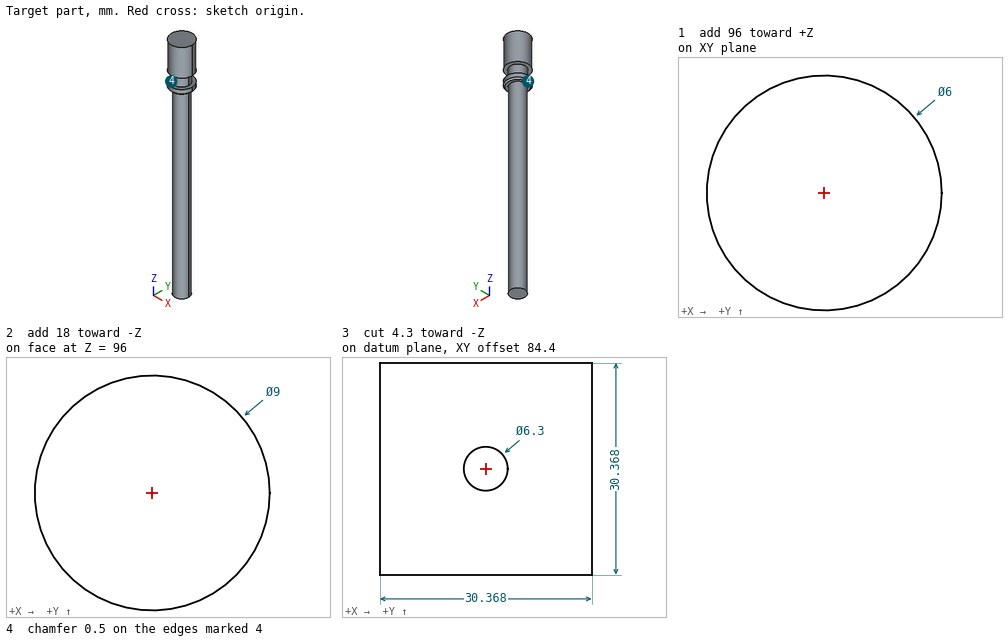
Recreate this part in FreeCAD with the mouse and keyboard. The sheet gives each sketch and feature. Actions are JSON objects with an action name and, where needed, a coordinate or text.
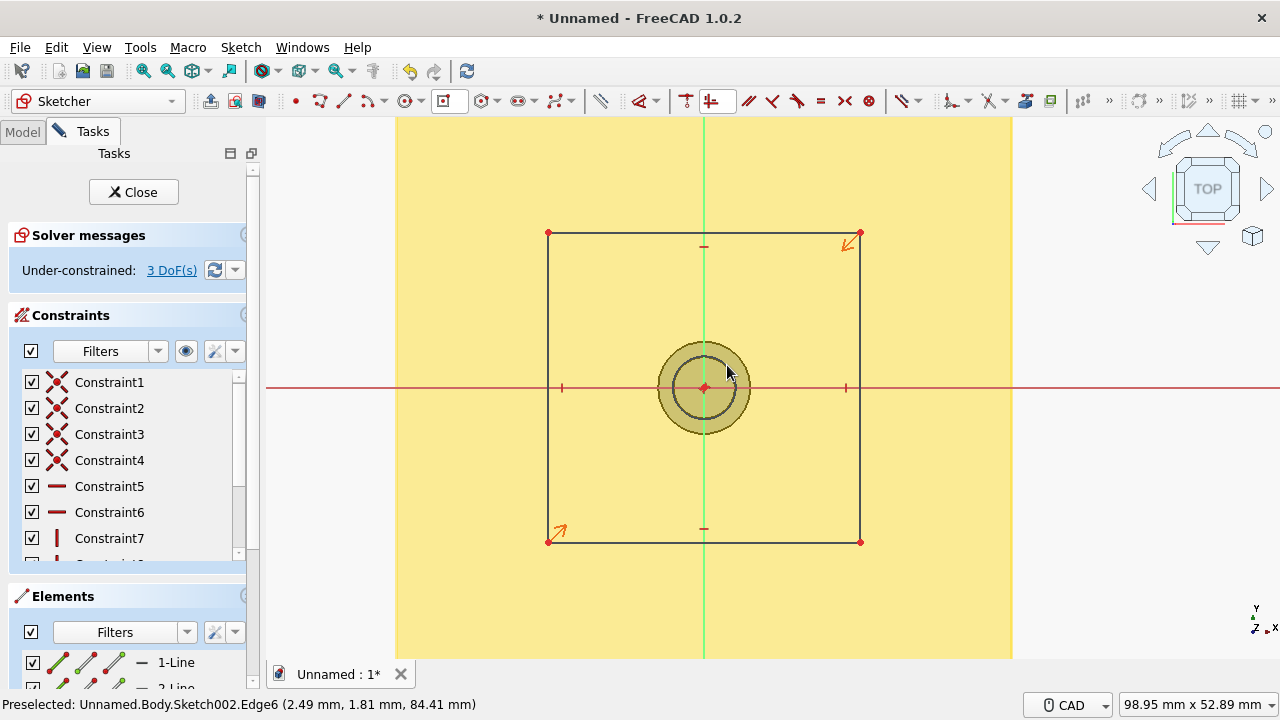
{"action": "left_click", "coordinate": [640, 102]}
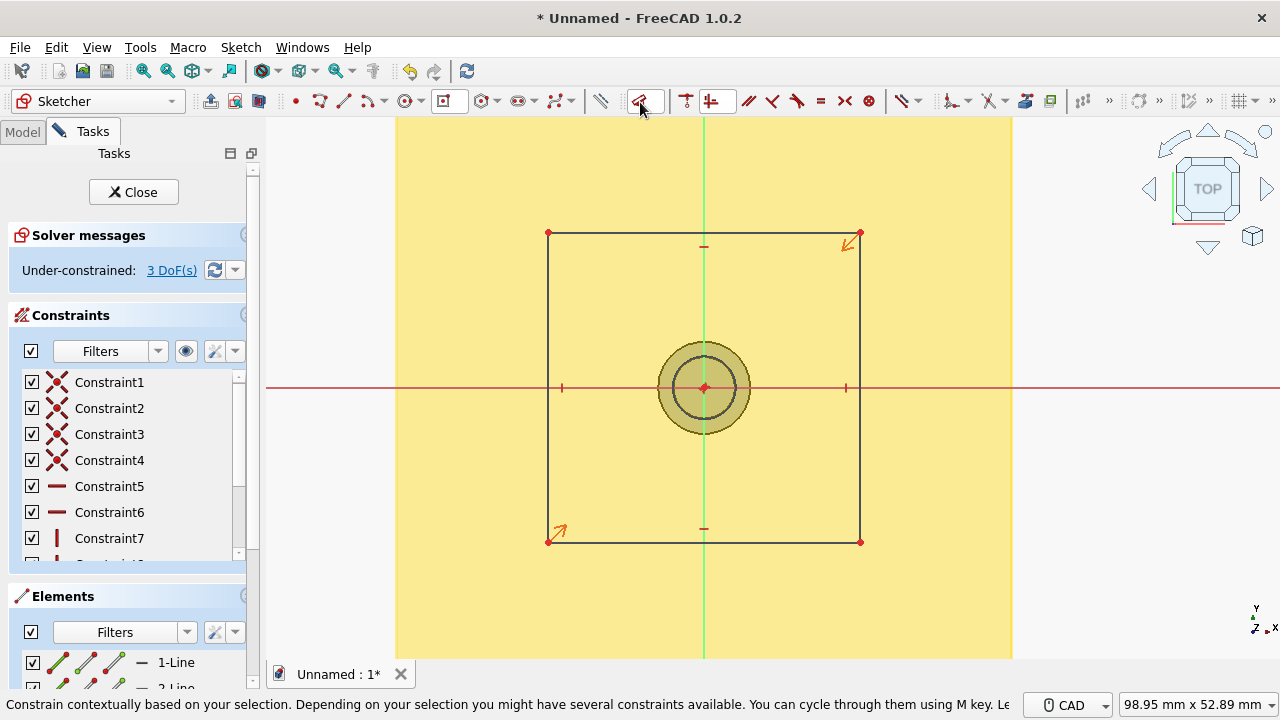
{"action": "left_click", "coordinate": [726, 365]}
{"action": "left_click", "coordinate": [748, 342]}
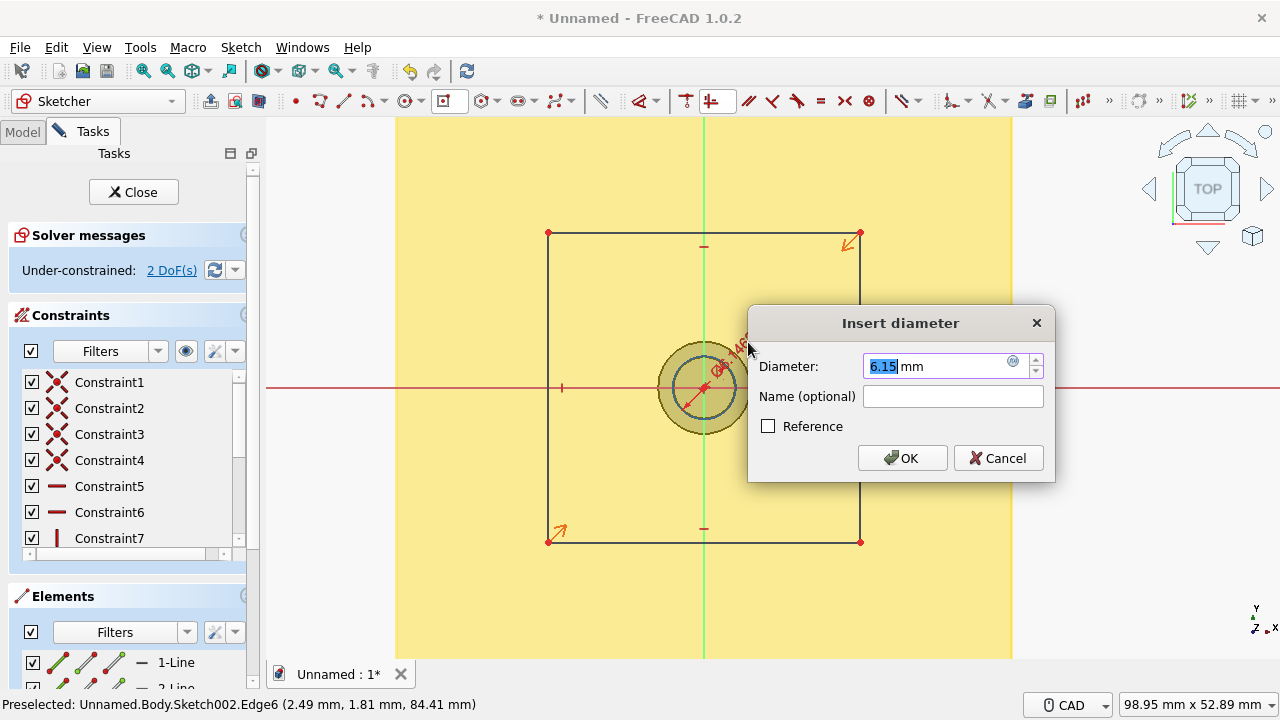
{"action": "type", "text": "6.3"}
{"action": "key", "text": "Return"}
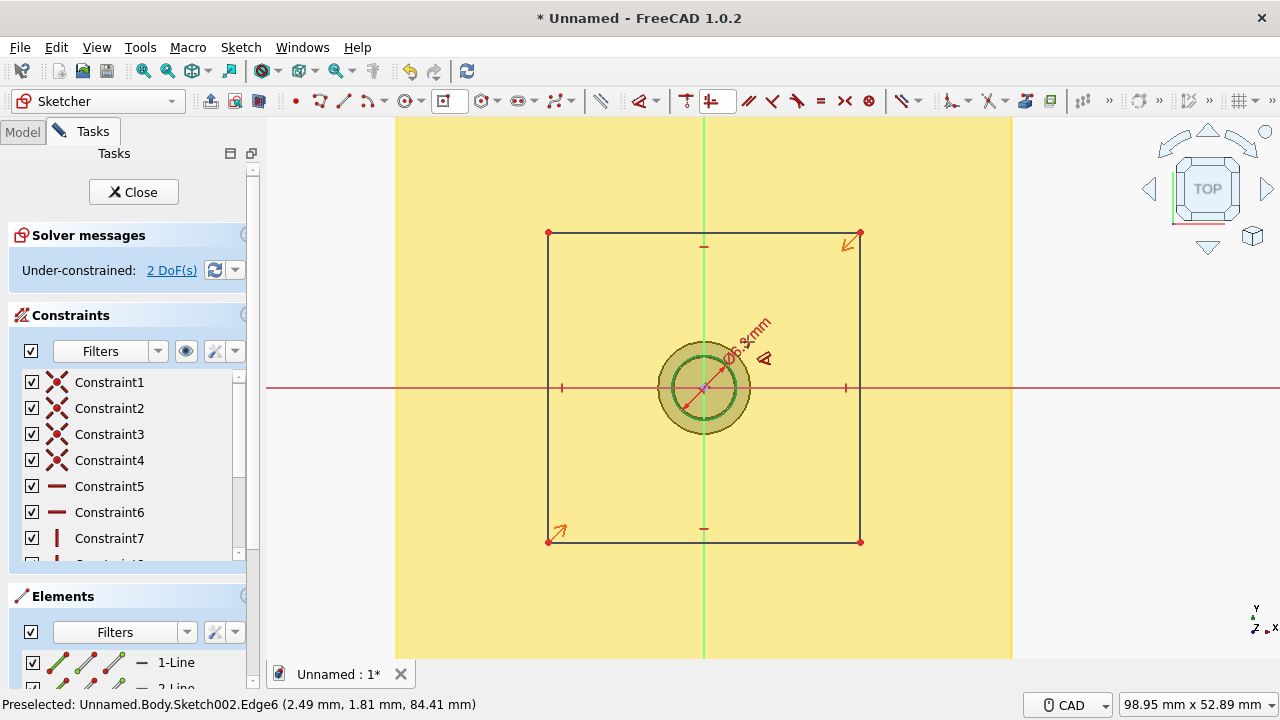
{"action": "left_click", "coordinate": [642, 543]}
{"action": "left_click", "coordinate": [633, 577]}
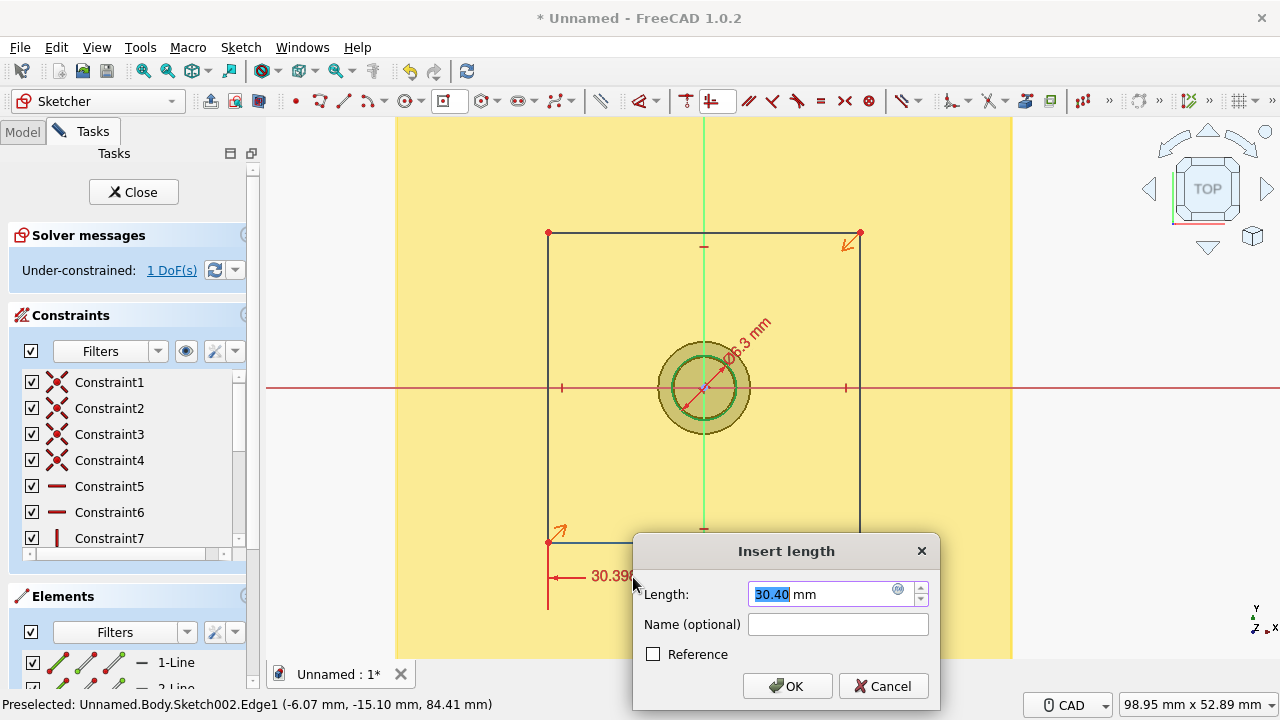
{"action": "type", "text": "30.368"}
{"action": "key", "text": "Return"}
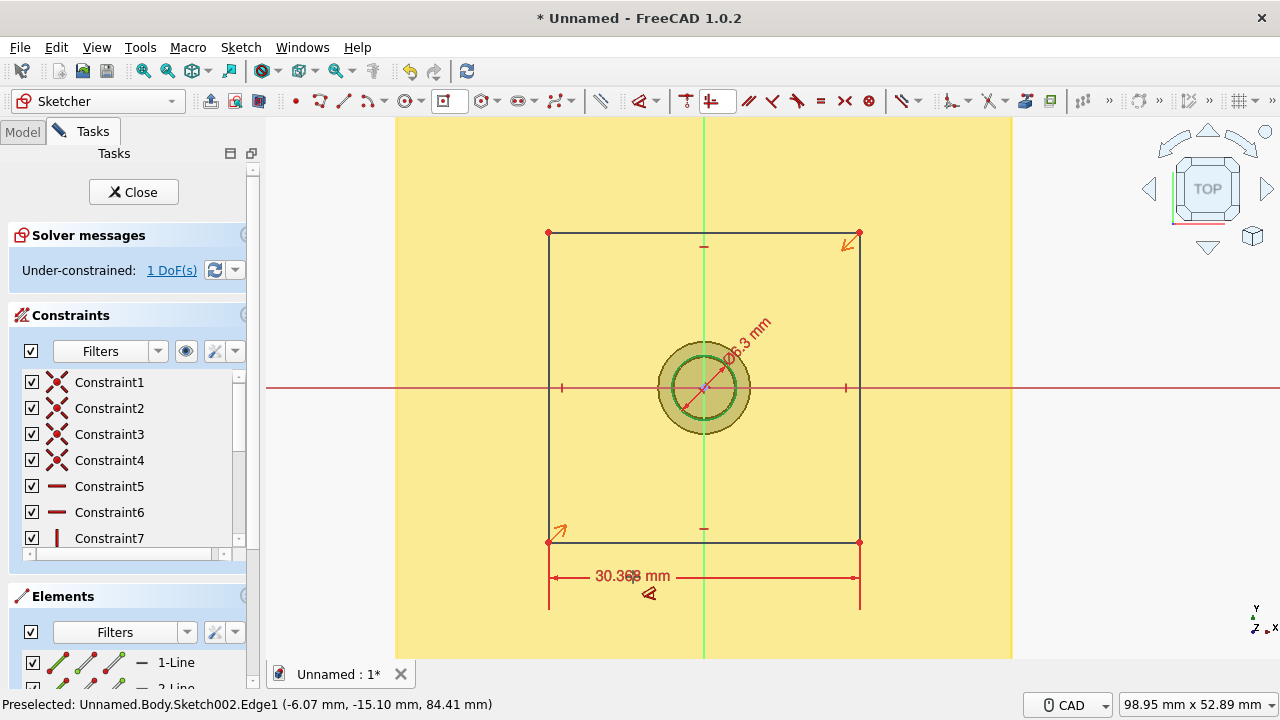
{"action": "left_click", "coordinate": [860, 450]}
{"action": "left_click", "coordinate": [894, 317]}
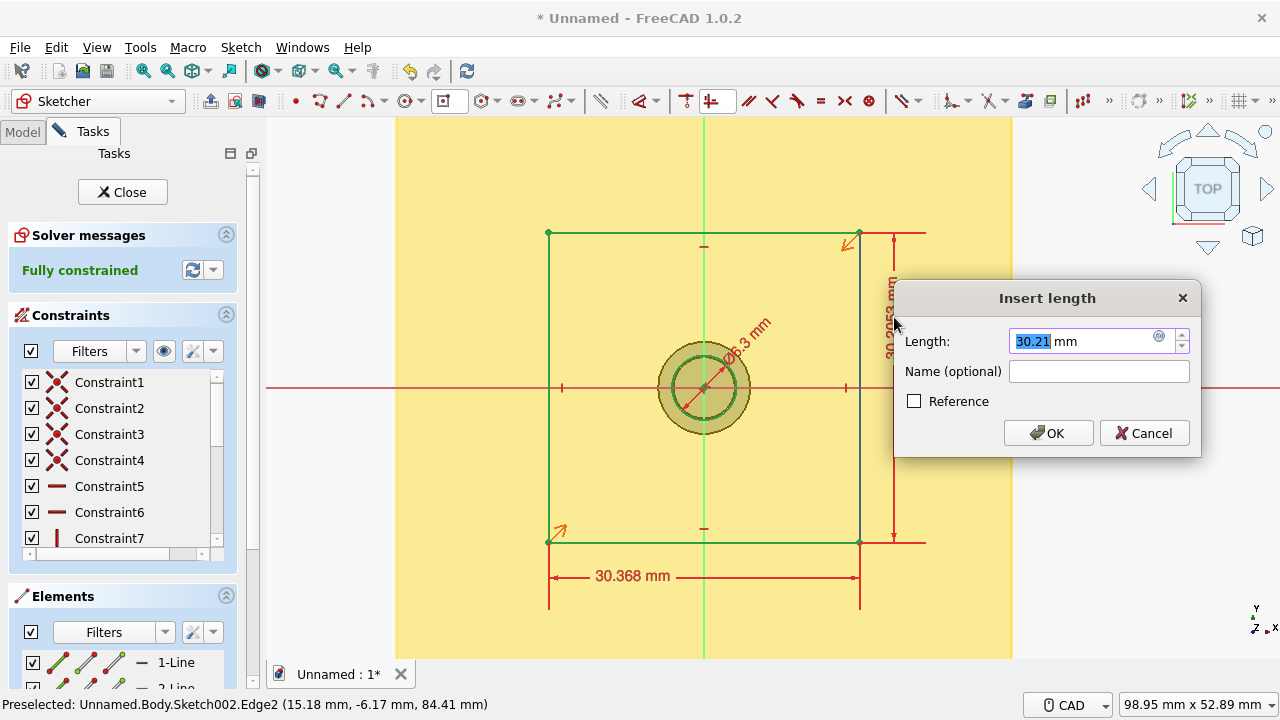
{"action": "type", "text": "30.368"}
{"action": "key", "text": "Return"}
{"action": "key", "text": "Escape"}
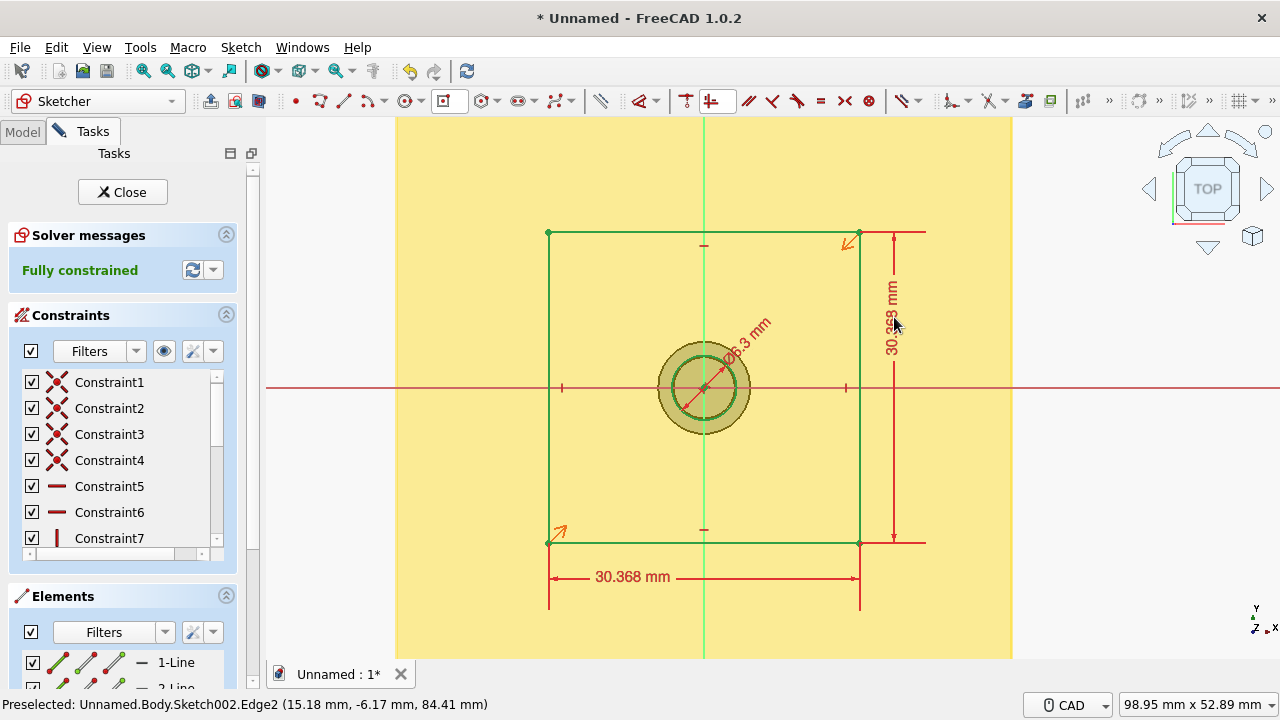
{"action": "left_click", "coordinate": [123, 192]}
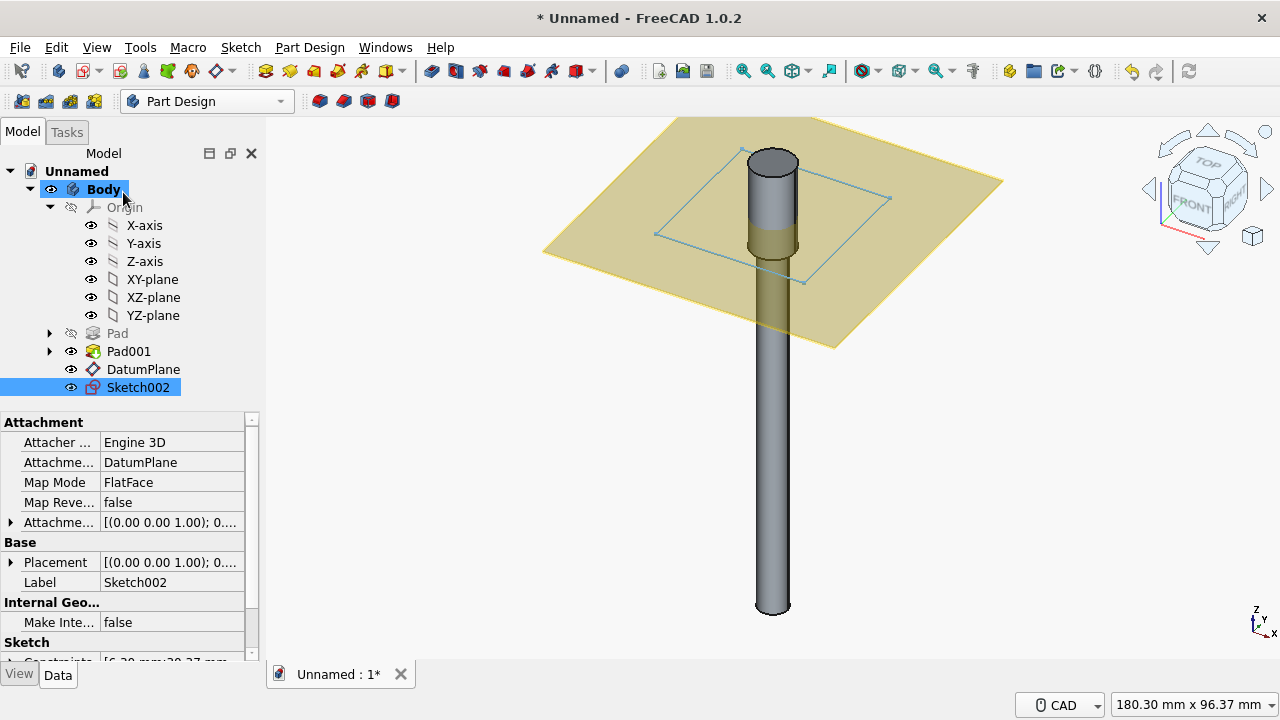
{"action": "left_click", "coordinate": [432, 72]}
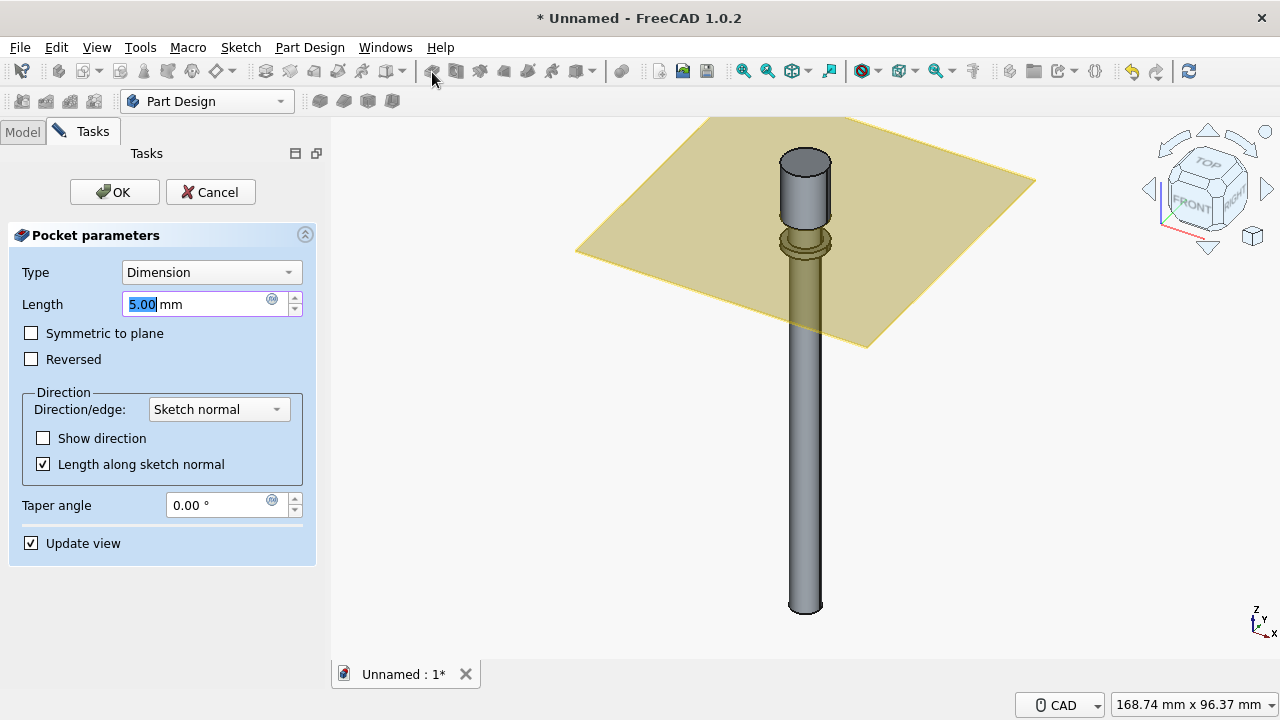
{"action": "type", "text": "4.3"}
{"action": "key", "text": "Tab"}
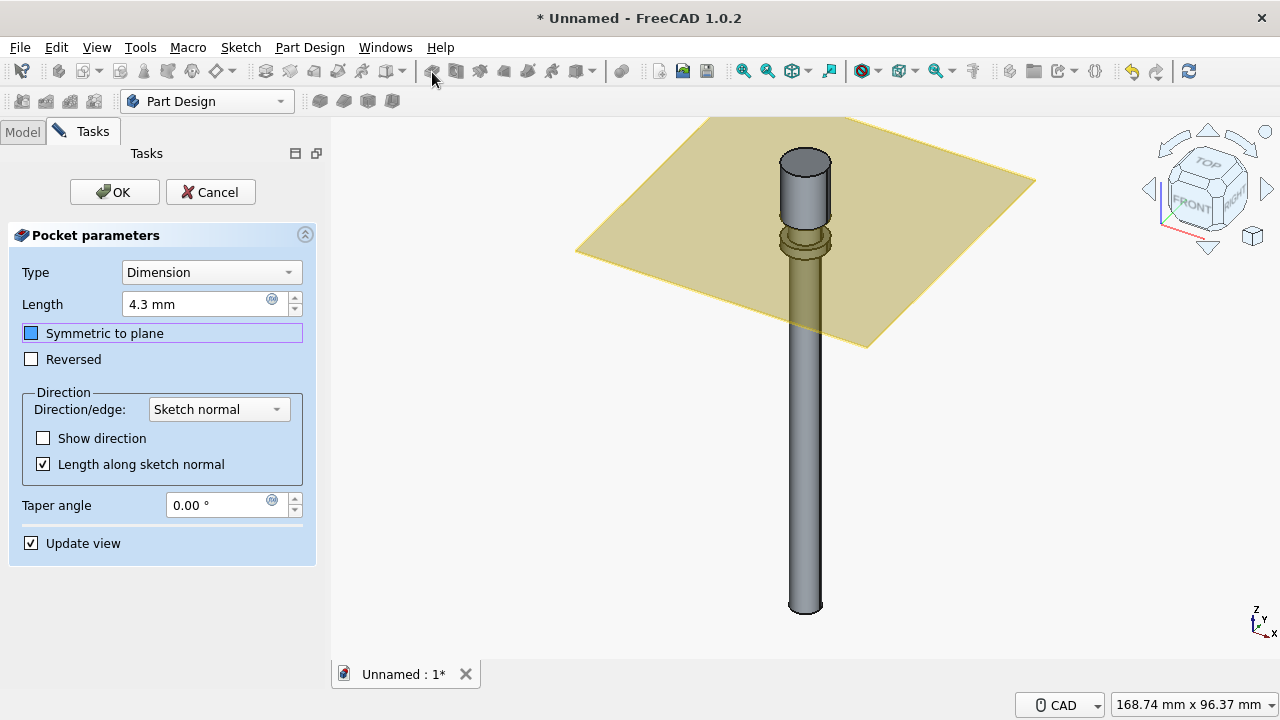
{"action": "left_click", "coordinate": [115, 192]}